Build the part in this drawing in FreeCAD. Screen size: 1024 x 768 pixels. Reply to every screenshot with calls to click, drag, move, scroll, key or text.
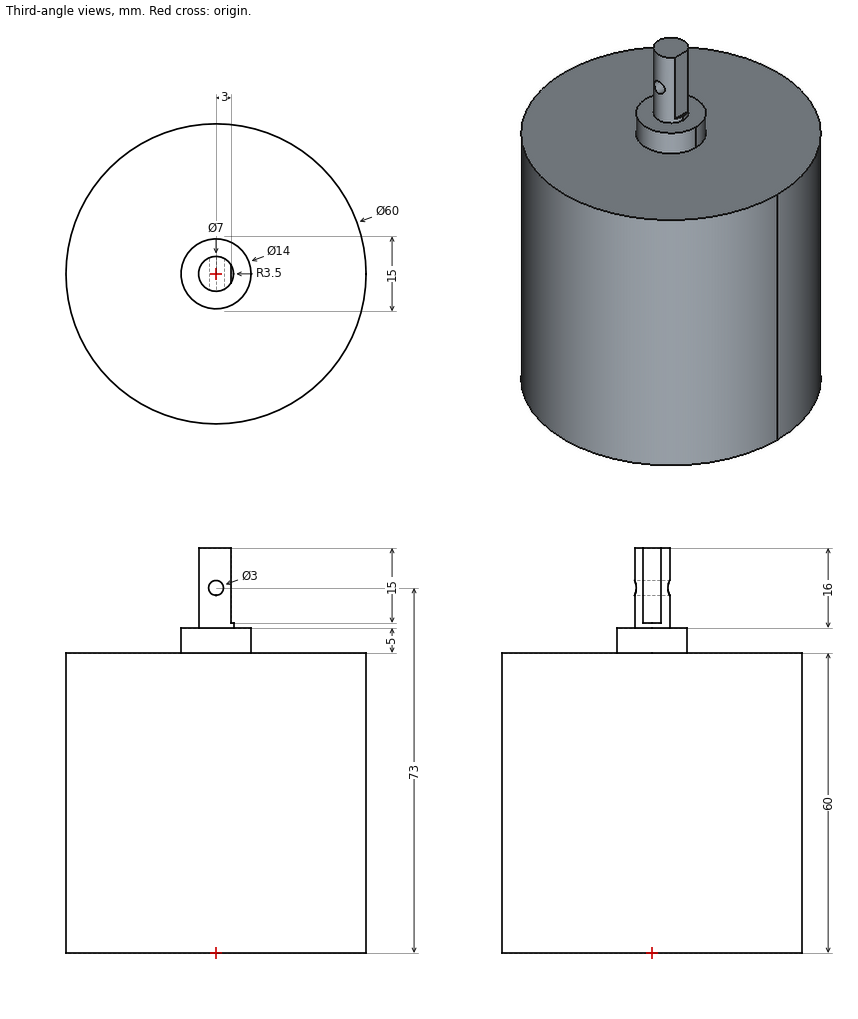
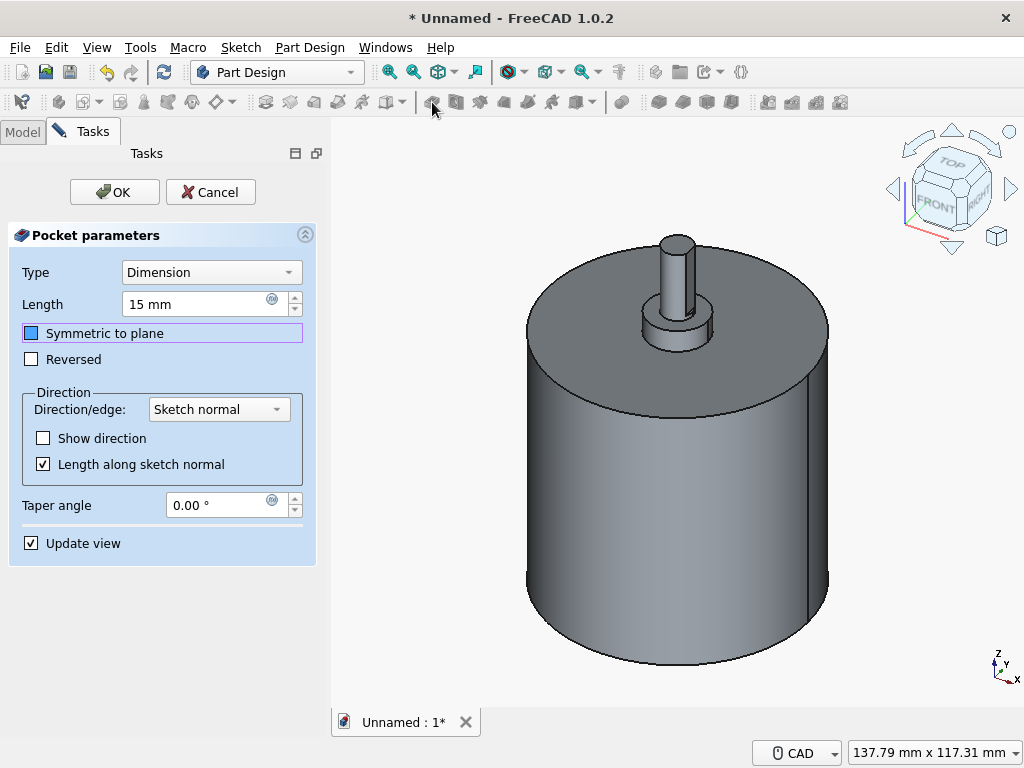
click(30, 333)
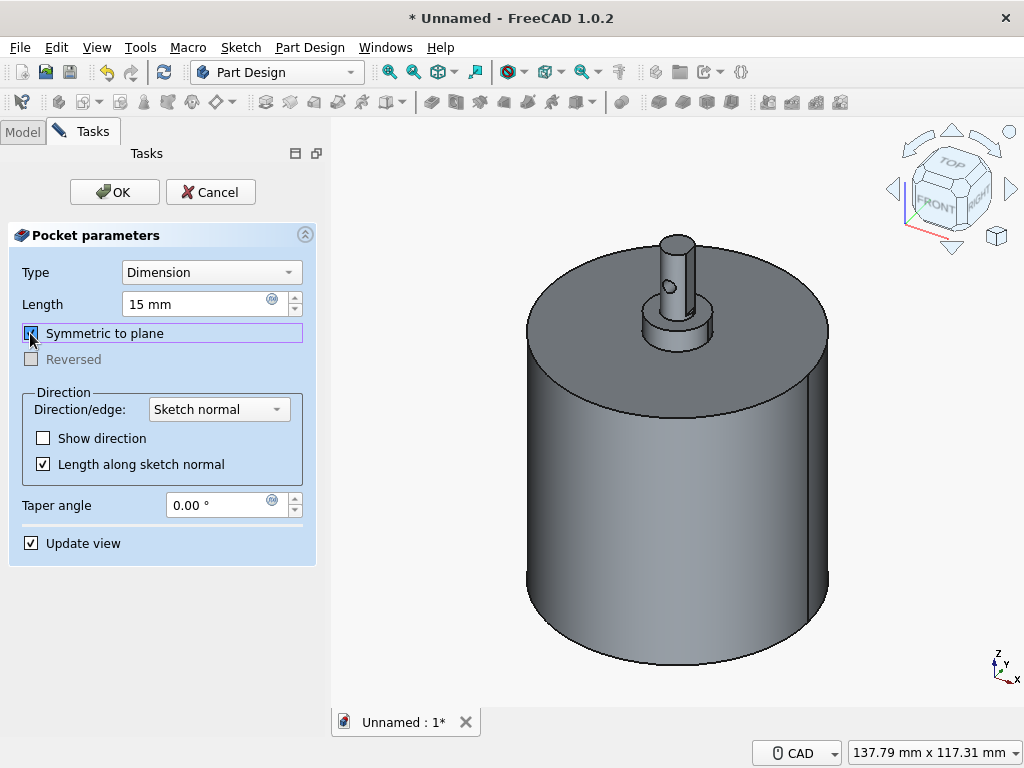
click(115, 192)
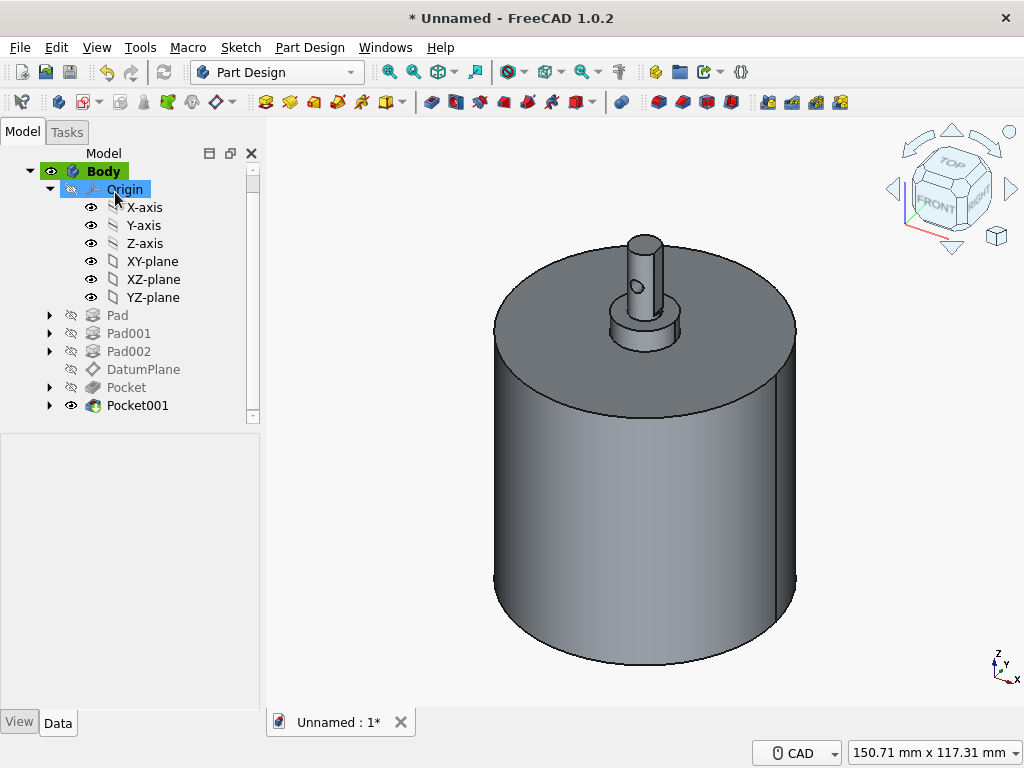
key(0)